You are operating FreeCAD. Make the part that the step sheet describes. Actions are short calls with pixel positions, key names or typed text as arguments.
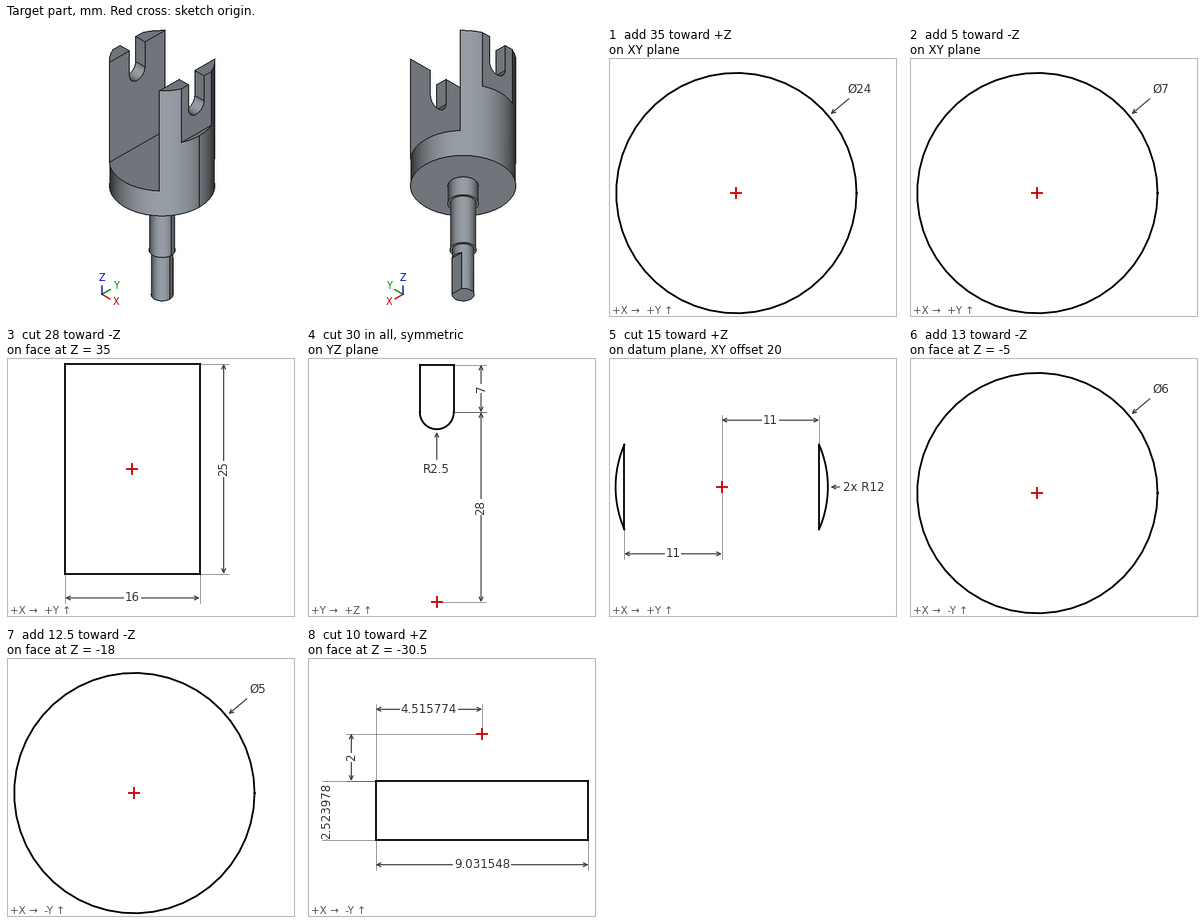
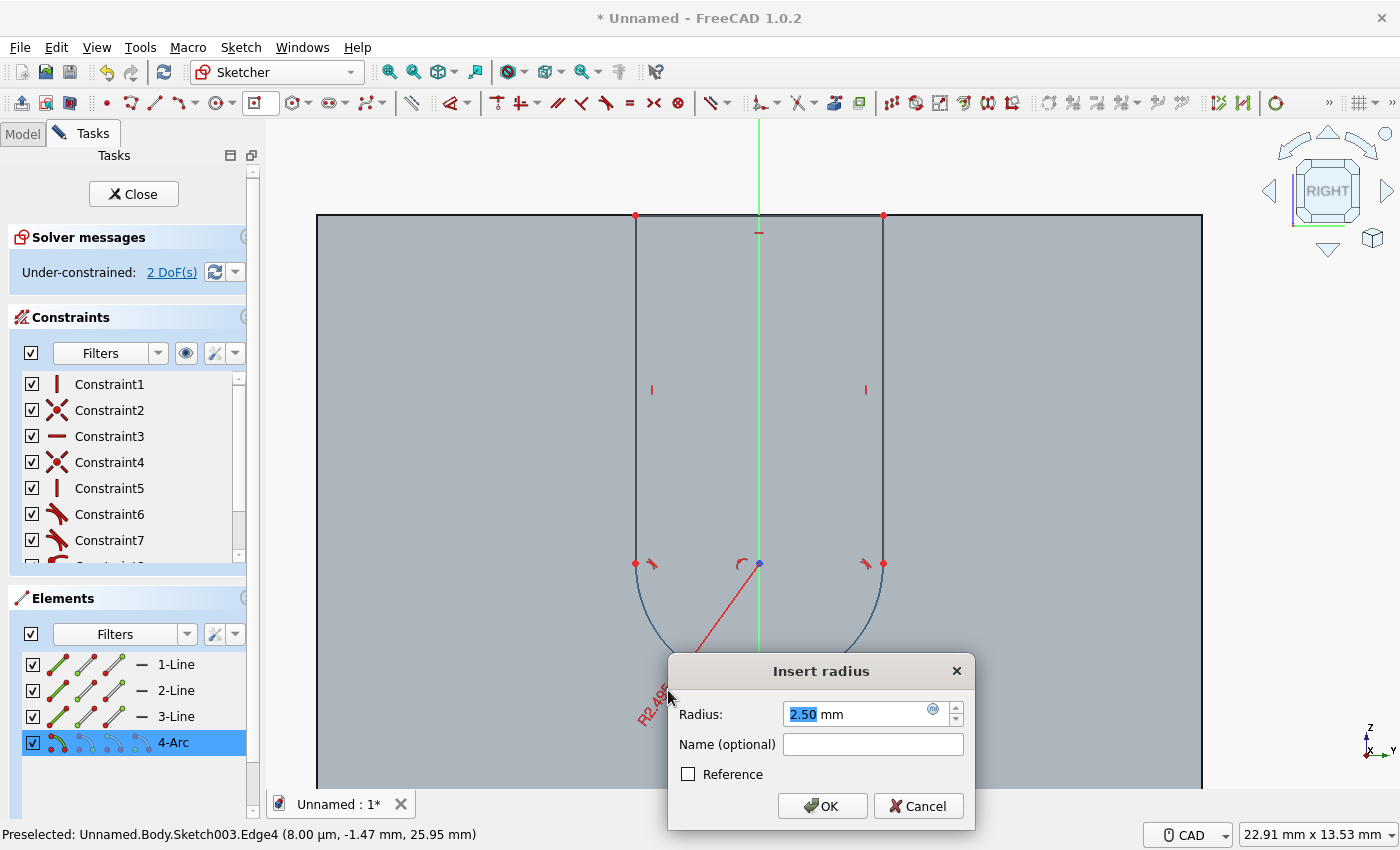
text(2.5)
key(Return)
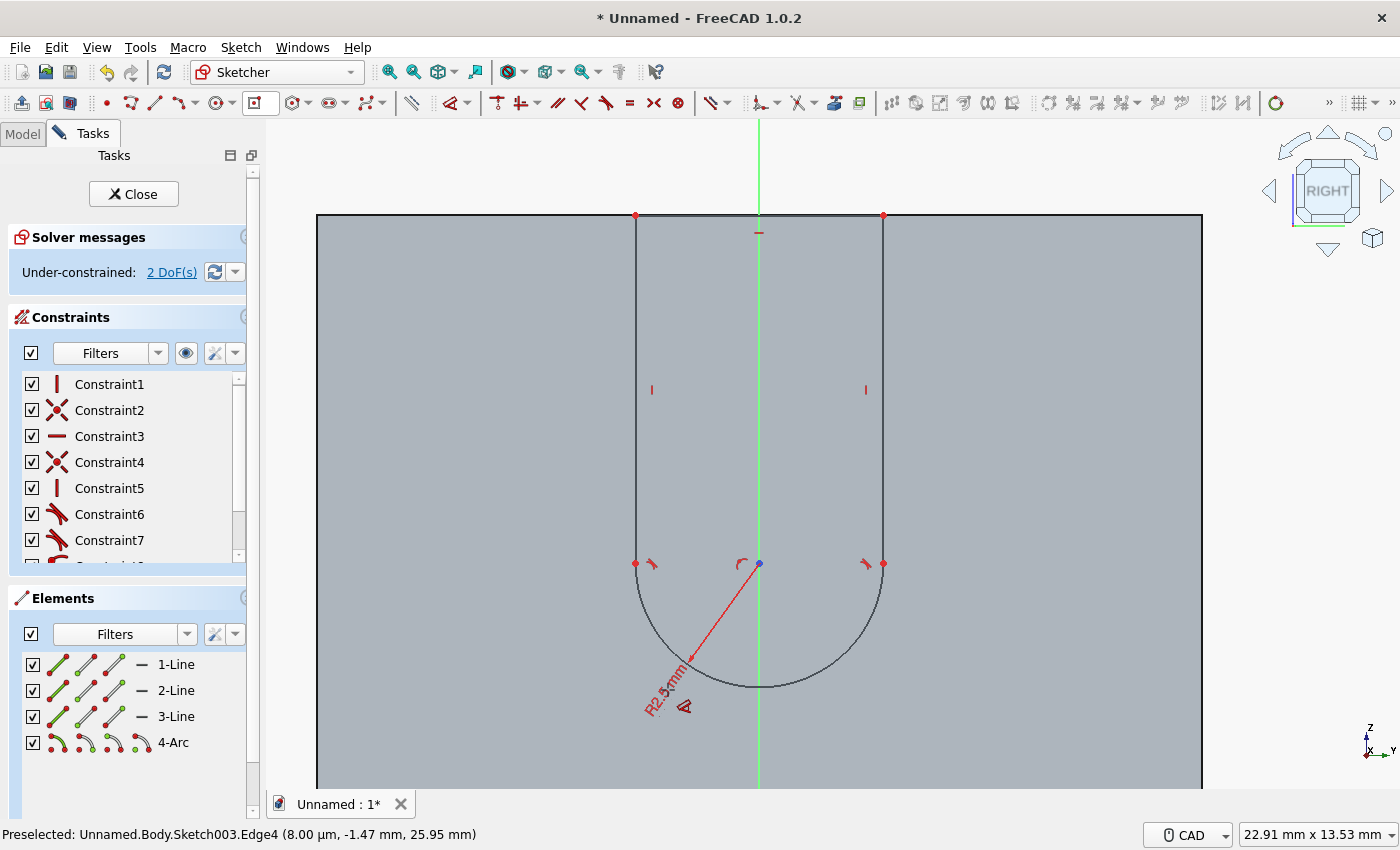
click(883, 459)
click(917, 390)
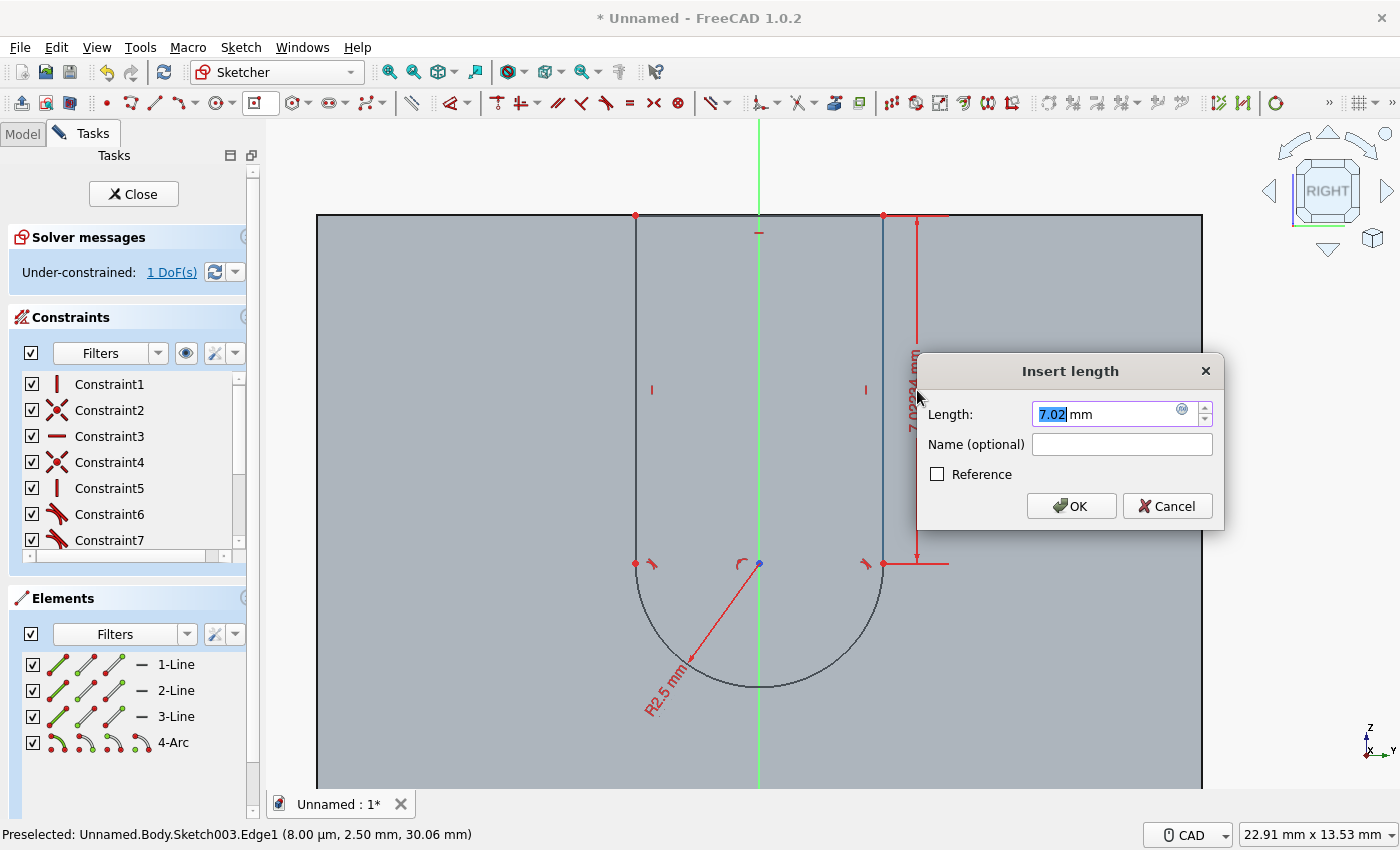
text(7)
key(Return)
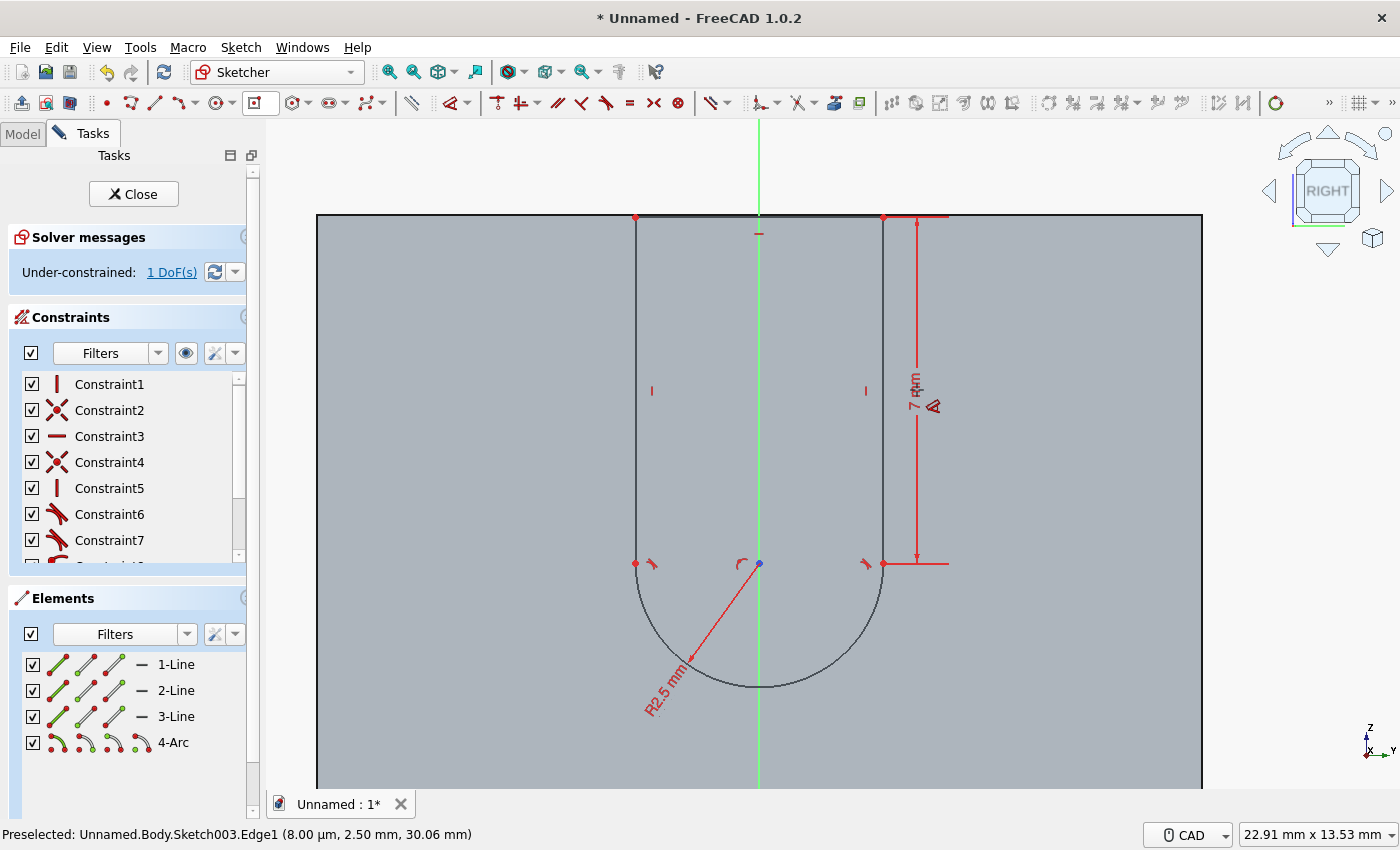
click(883, 564)
click(917, 662)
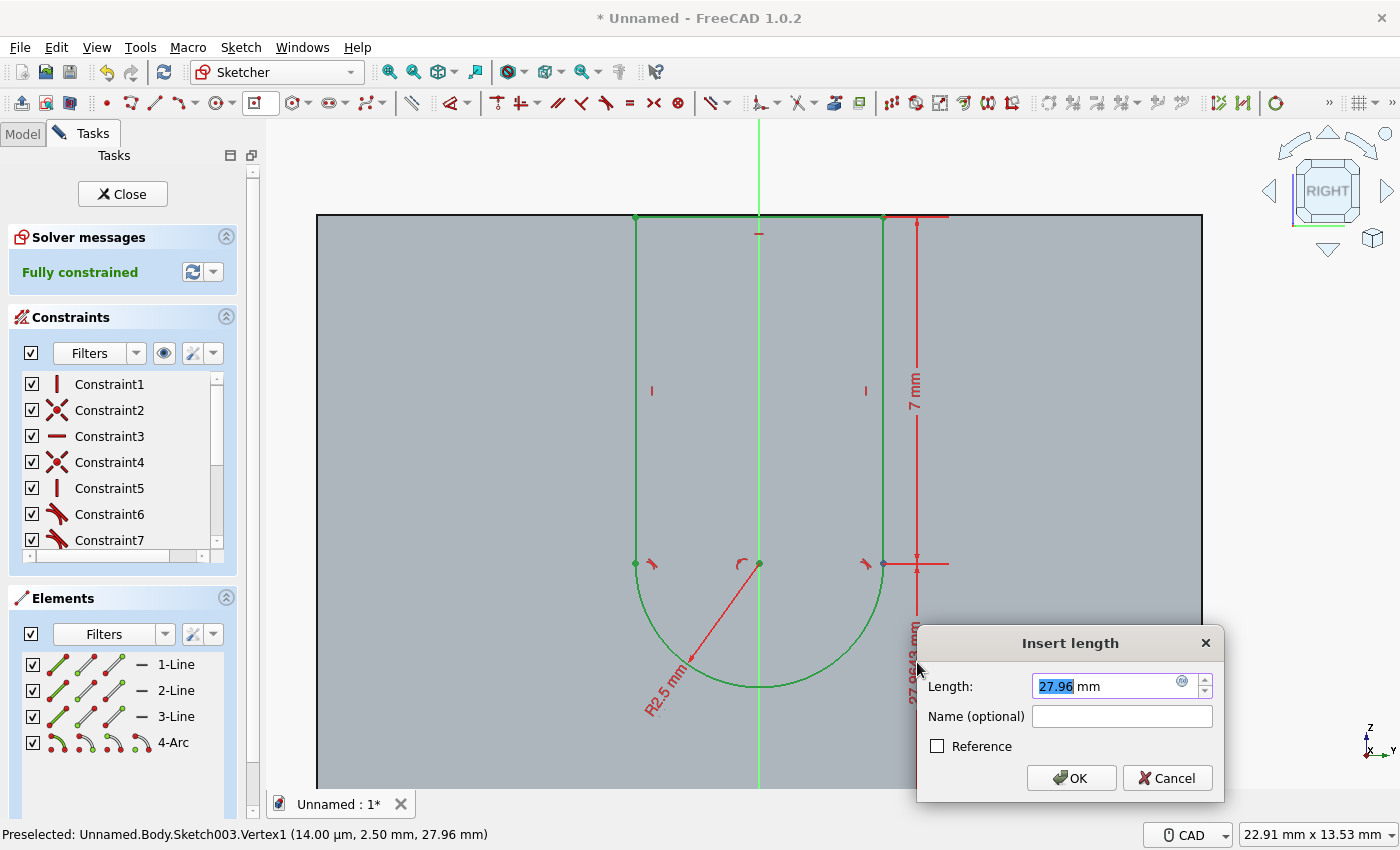
text(28)
key(Return)
key(Escape)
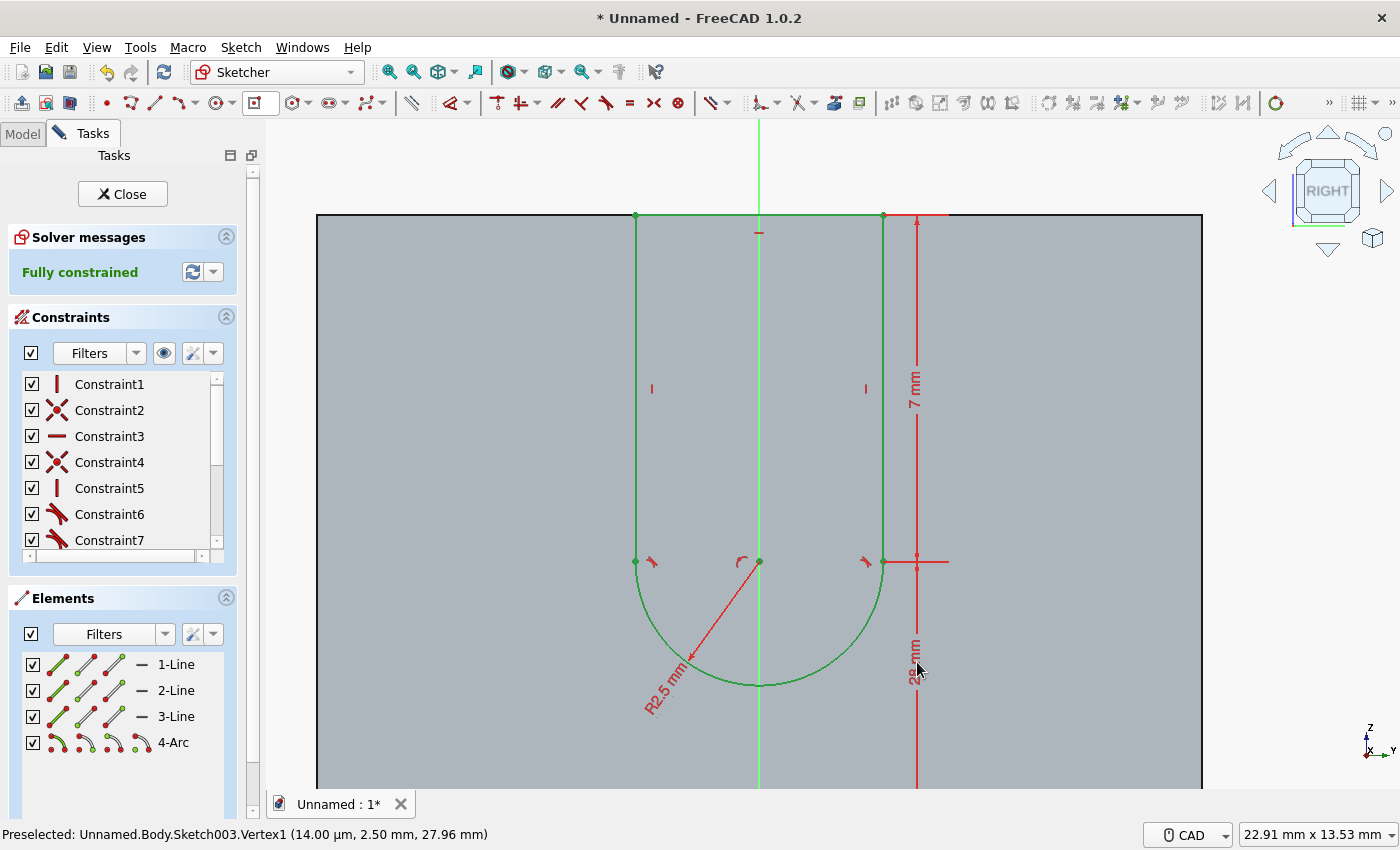
click(123, 194)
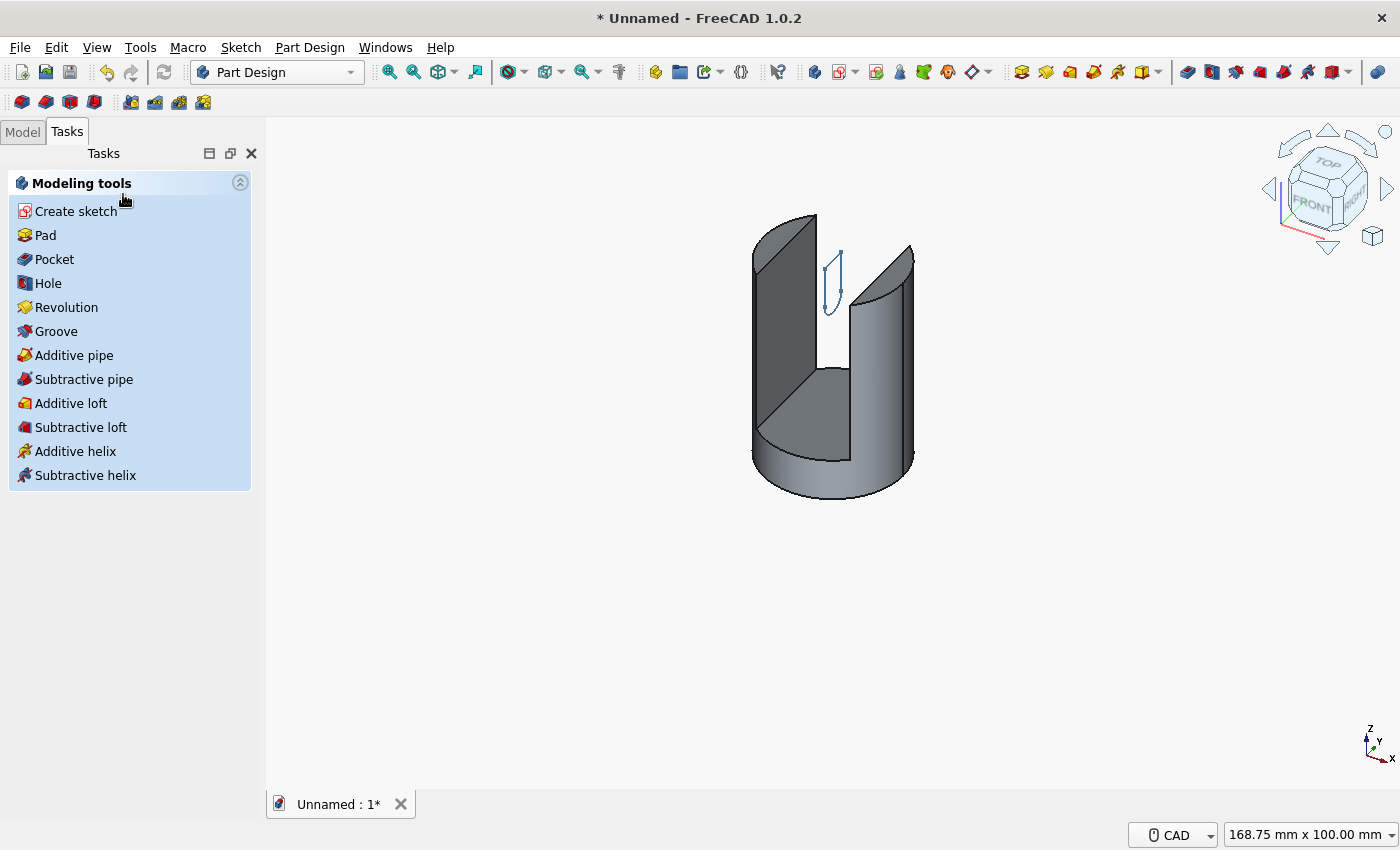
click(1188, 72)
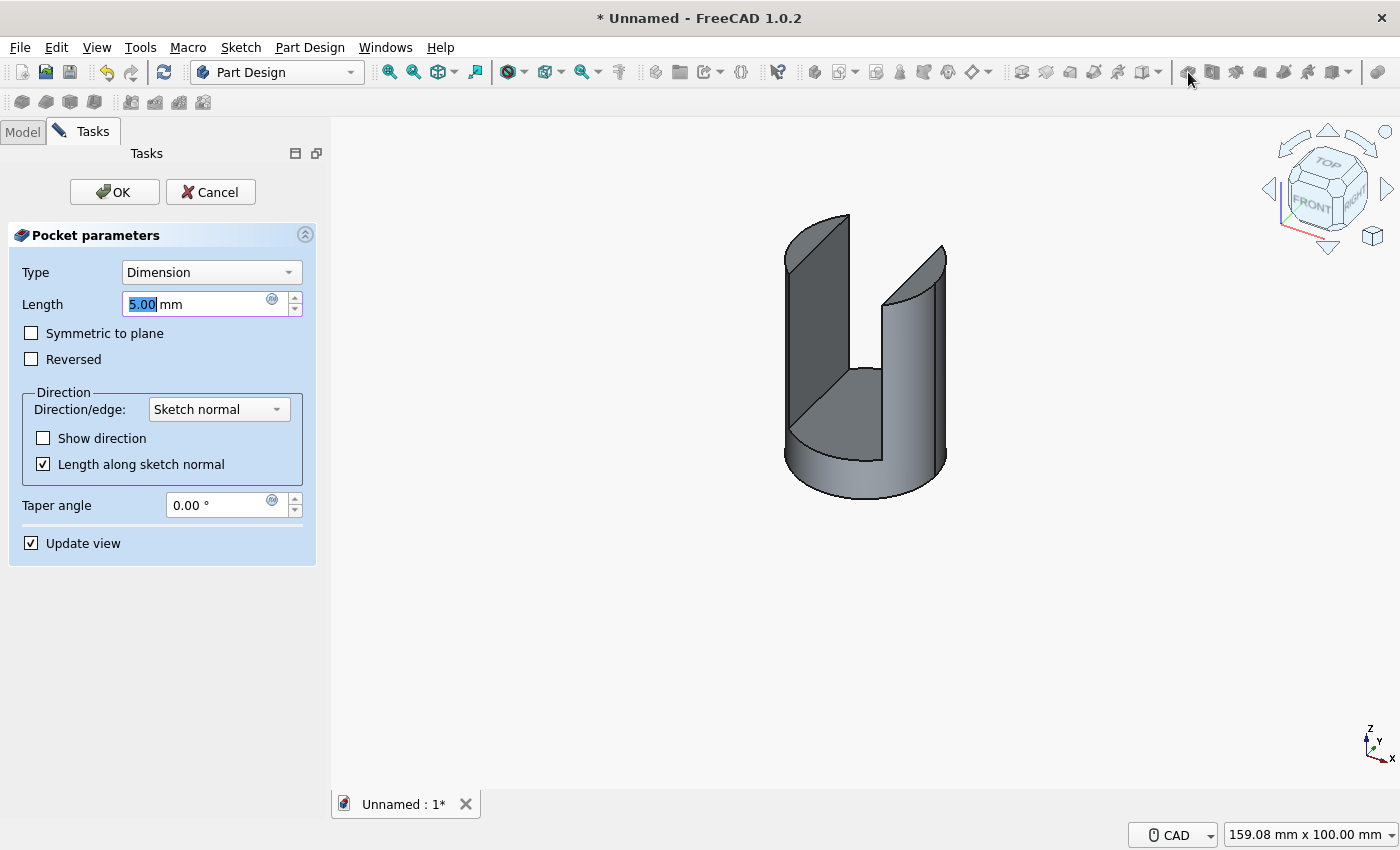
text(30)
key(Tab)